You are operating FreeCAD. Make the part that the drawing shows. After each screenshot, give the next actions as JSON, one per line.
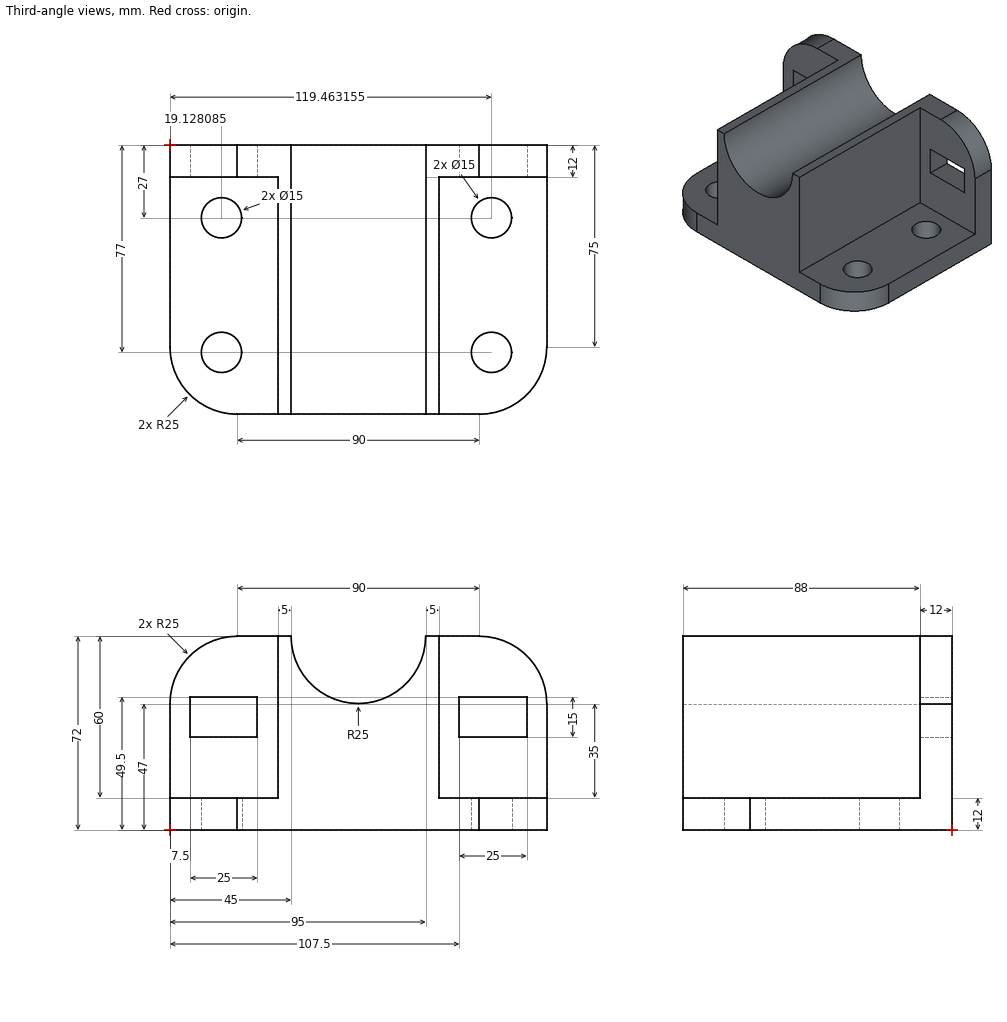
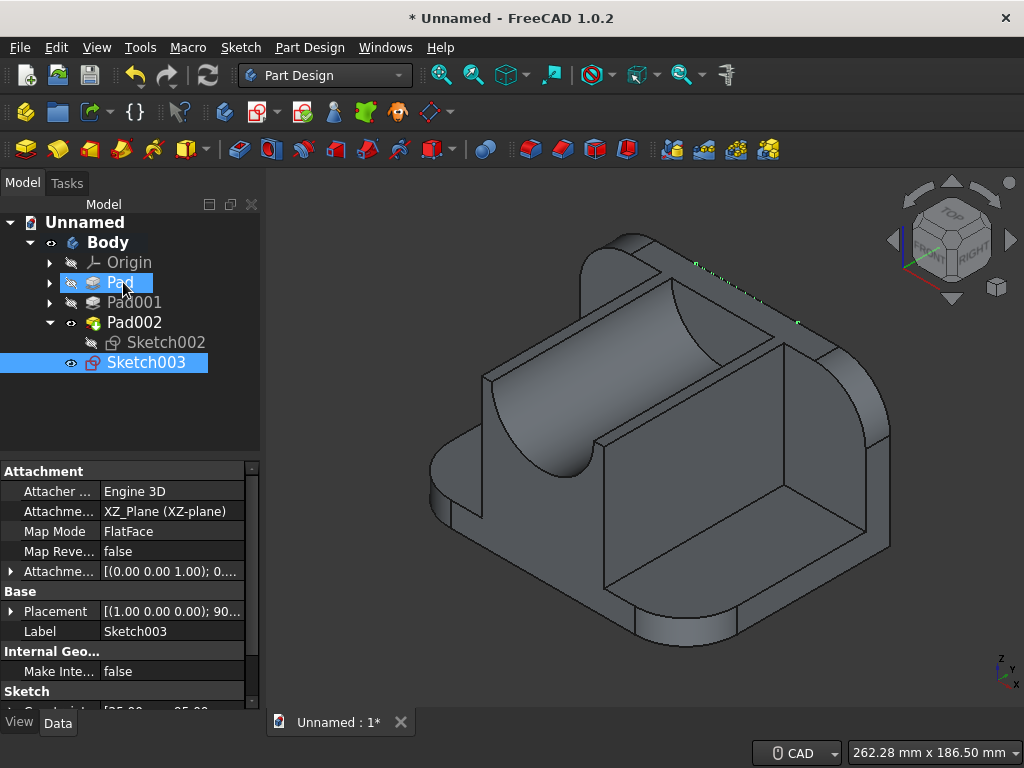
{"action": "left_click", "coordinate": [240, 150]}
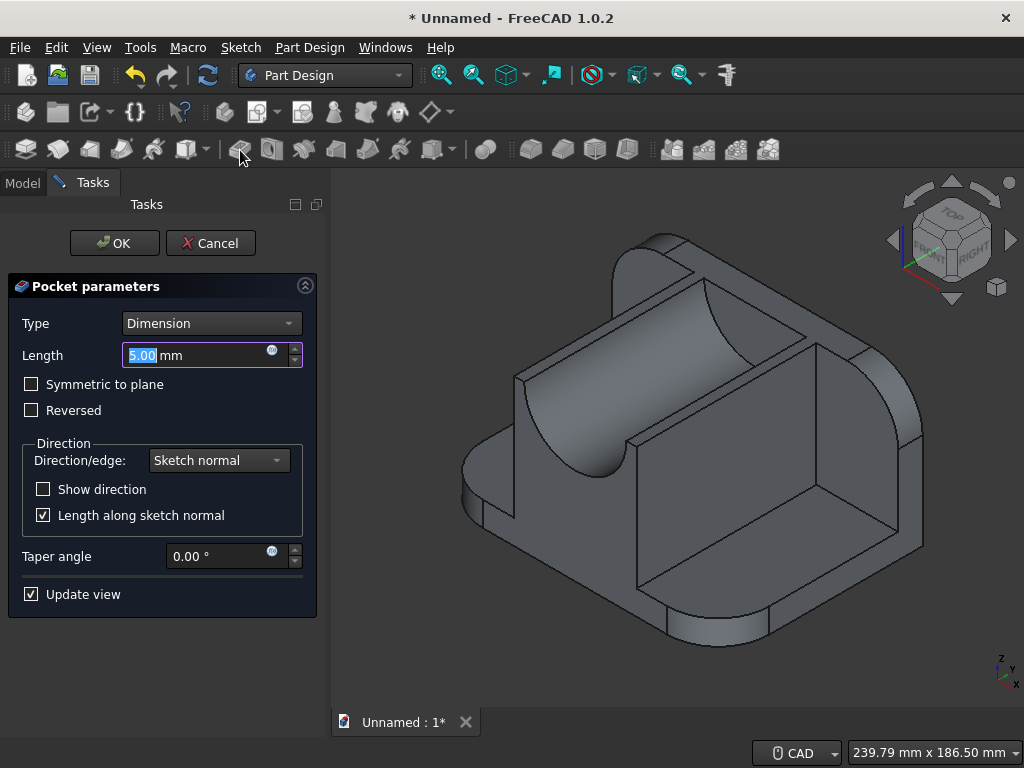
{"action": "type", "text": "12"}
{"action": "key", "text": "Tab"}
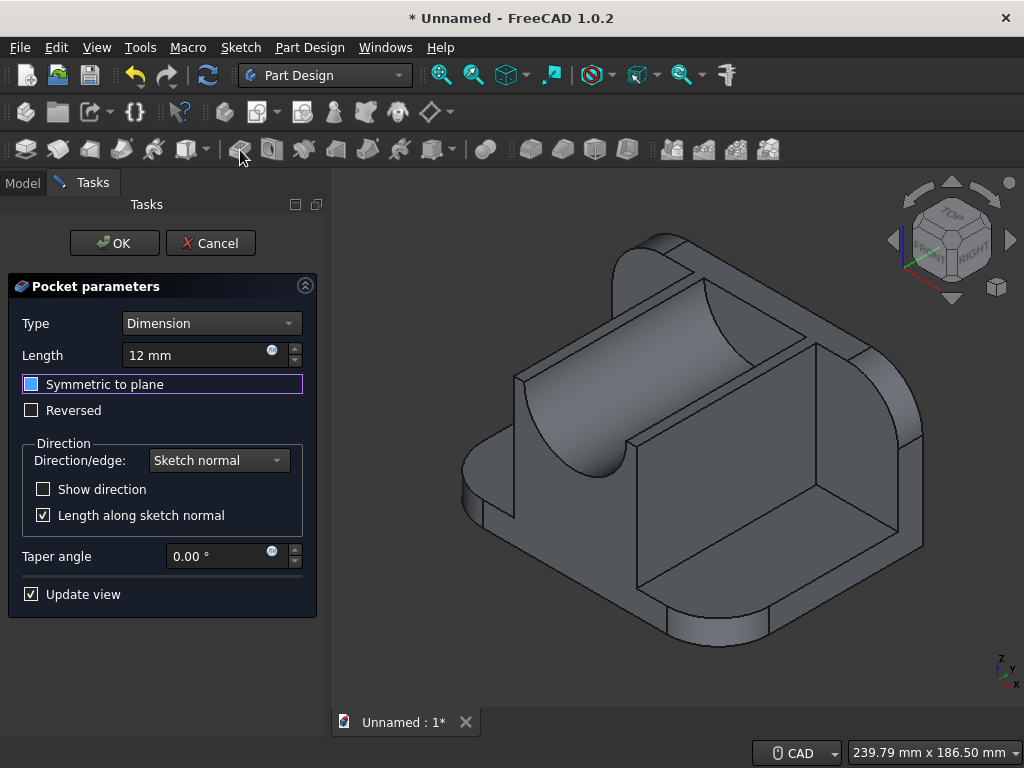
{"action": "left_click", "coordinate": [30, 410]}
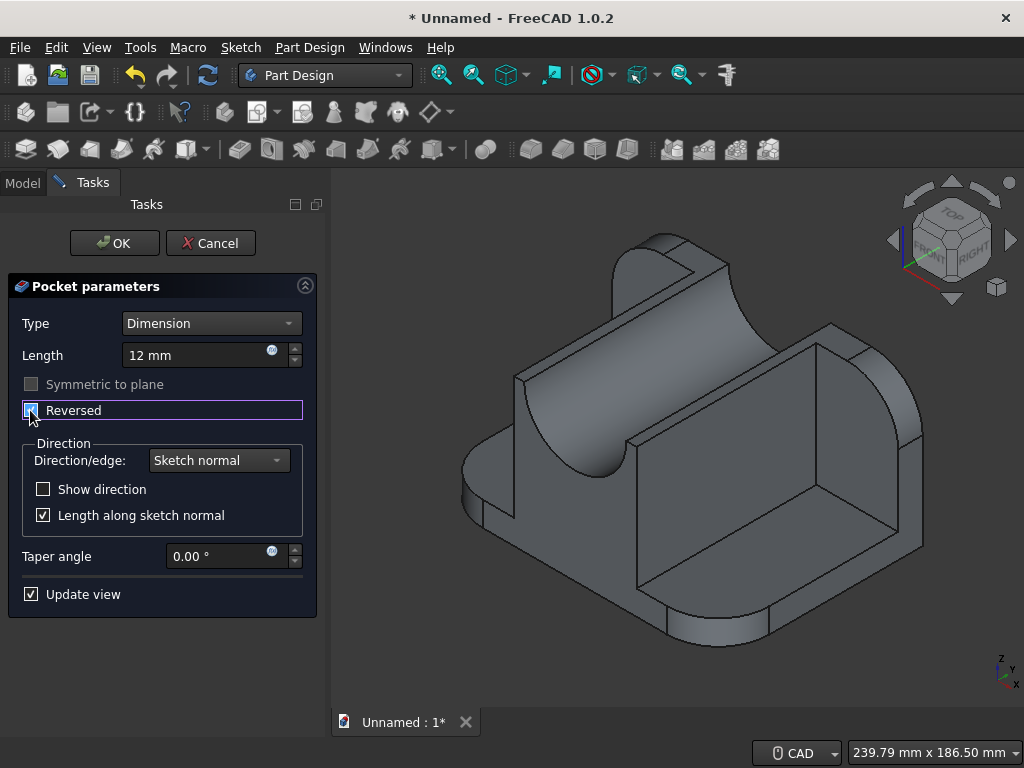
{"action": "left_click", "coordinate": [115, 243]}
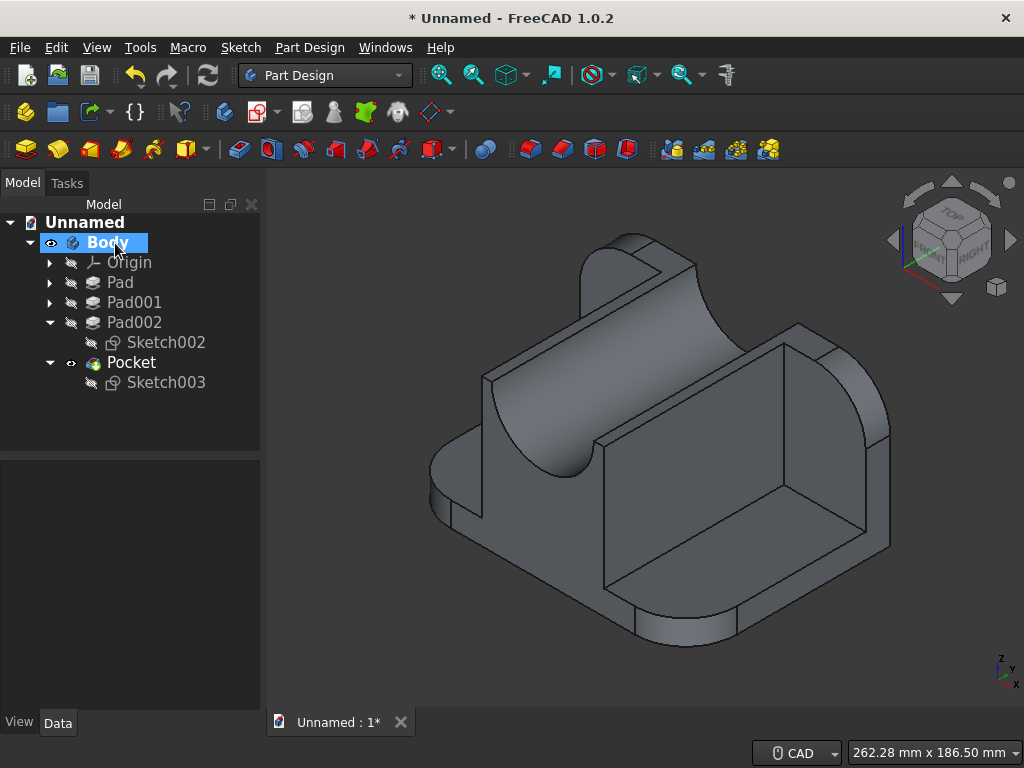
{"action": "key", "text": "1"}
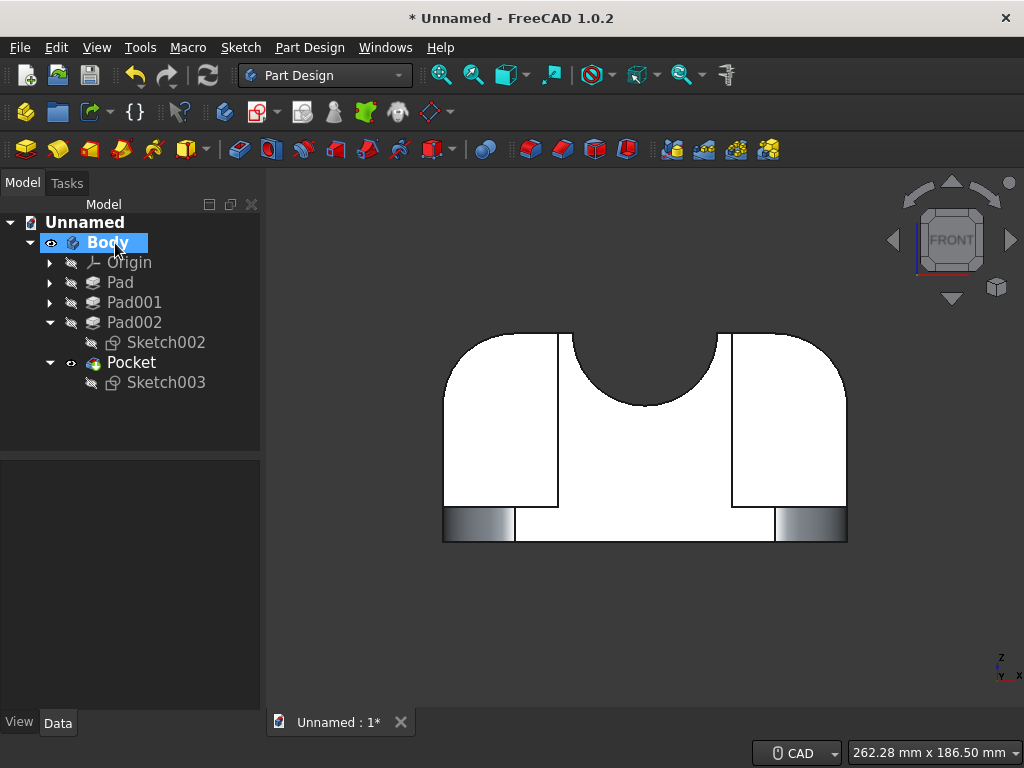
{"action": "left_click", "coordinate": [500, 419]}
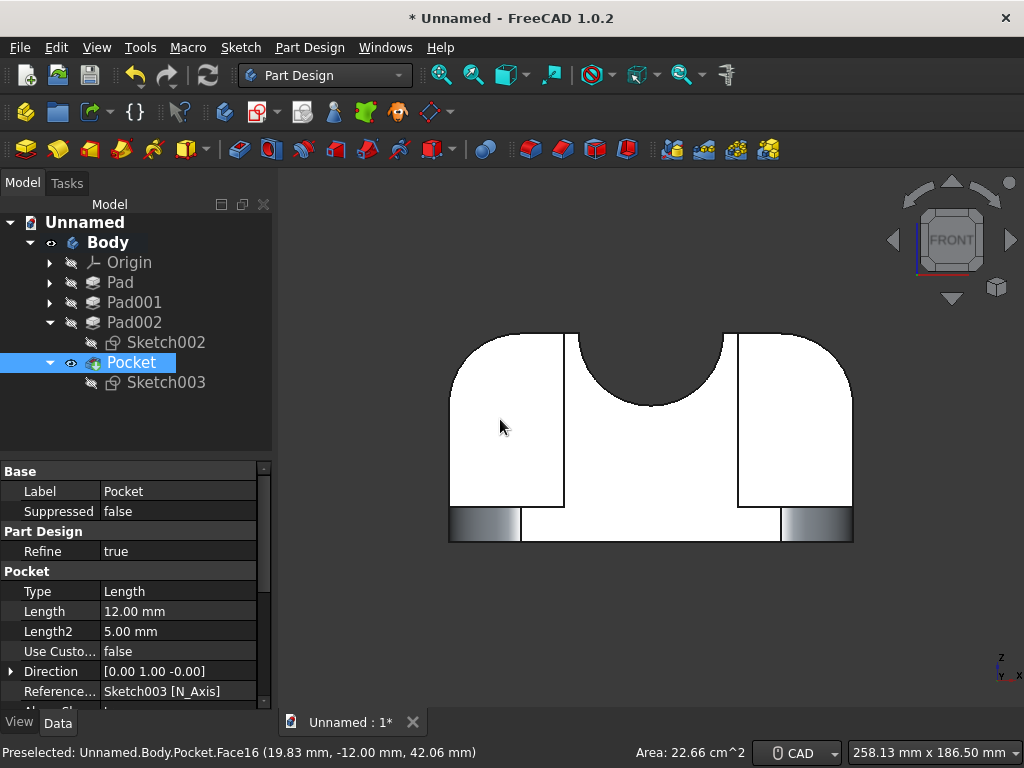
{"action": "left_click", "coordinate": [258, 112]}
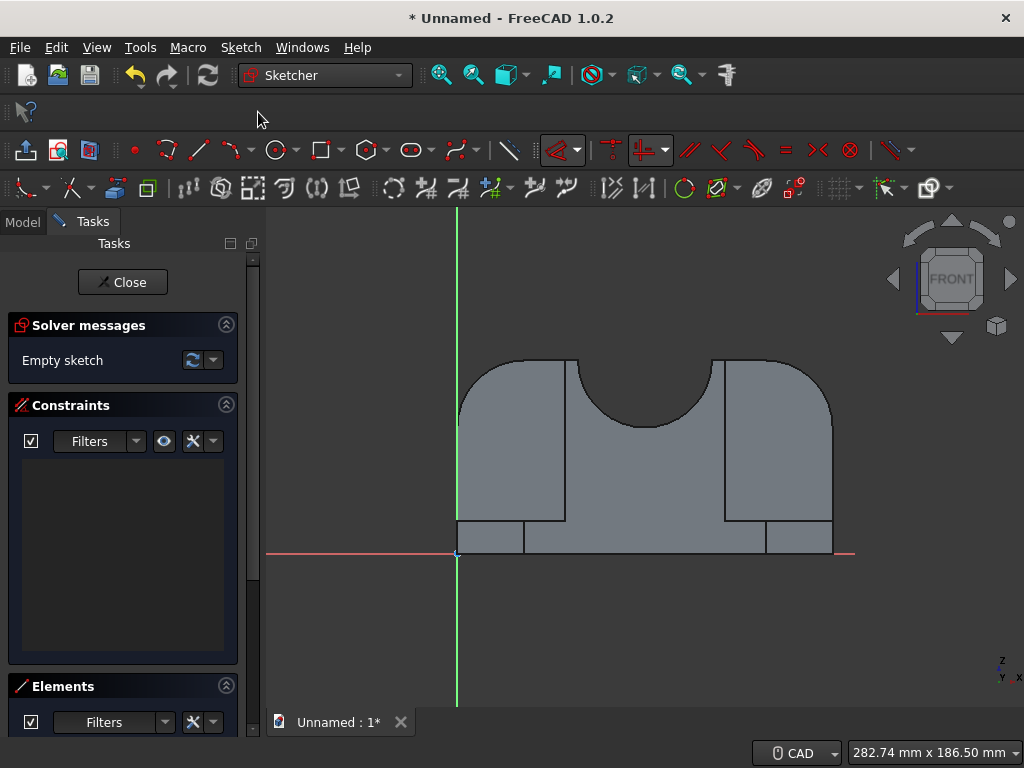
{"action": "scroll", "coordinate": [819, 438], "scroll_direction": "up", "scroll_amount": 9}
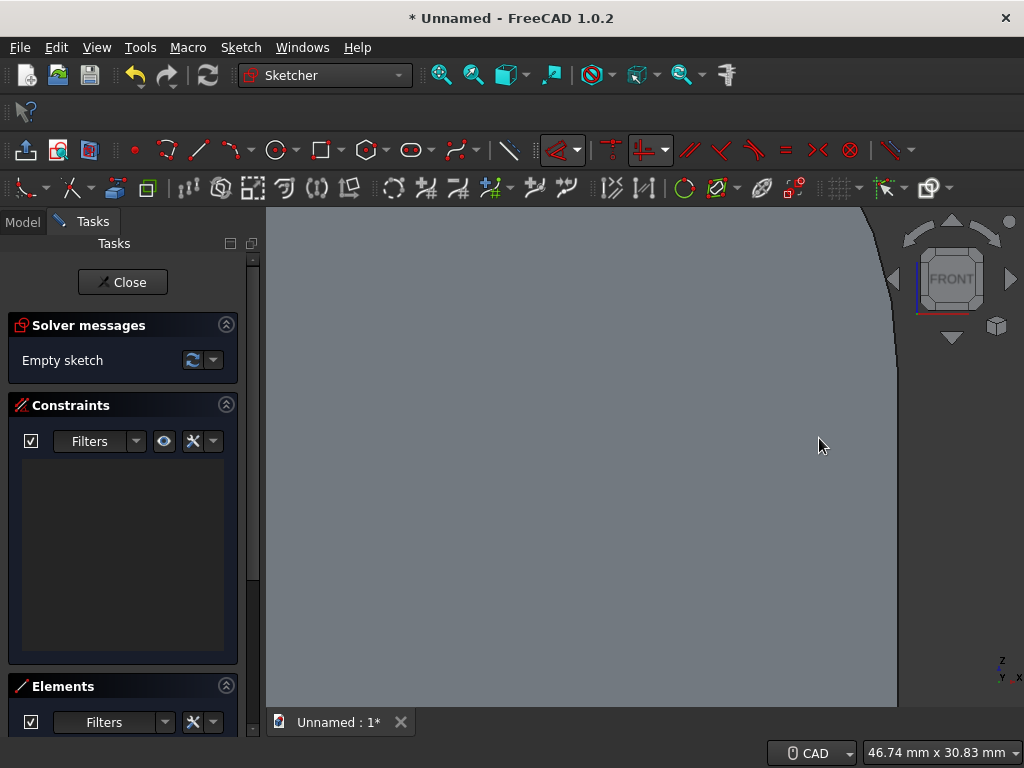
{"action": "key", "text": "g r"}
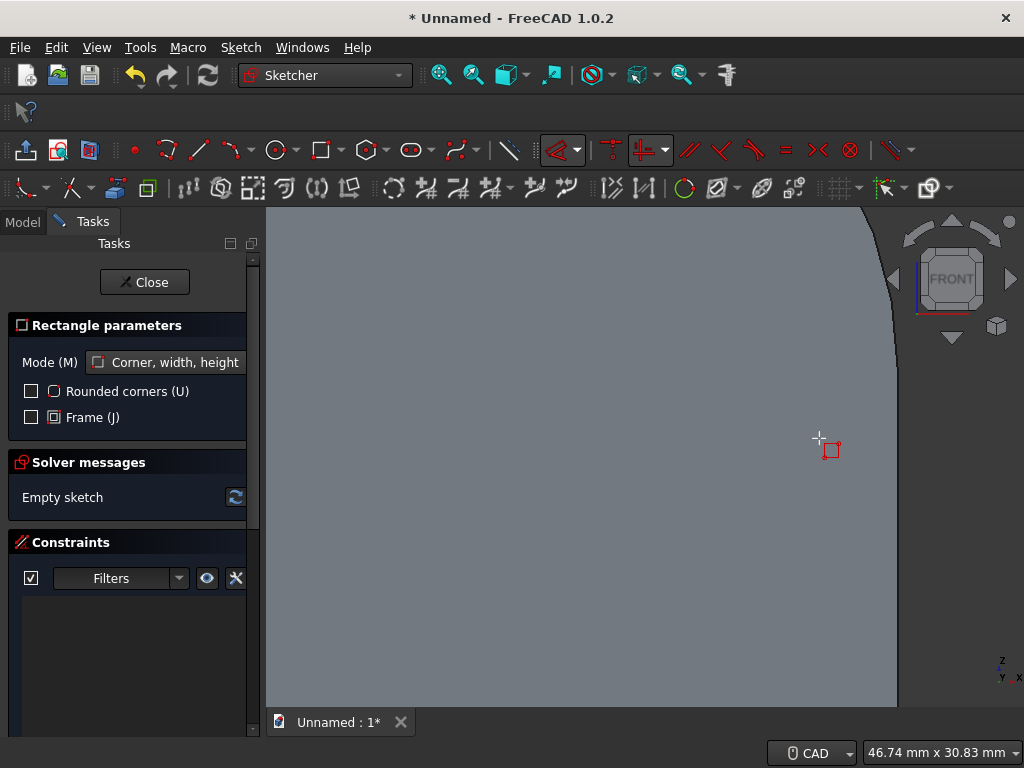
{"action": "left_click", "coordinate": [371, 332]}
{"action": "left_click", "coordinate": [776, 575]}
{"action": "key", "text": "Escape"}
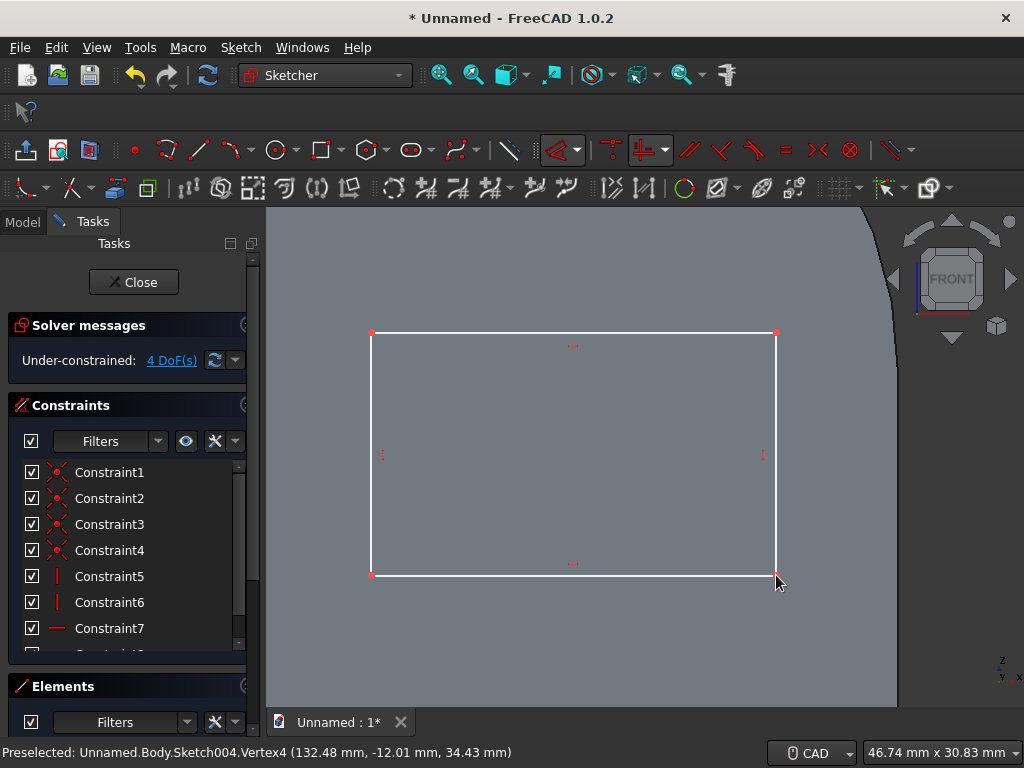
{"action": "left_click", "coordinate": [371, 406]}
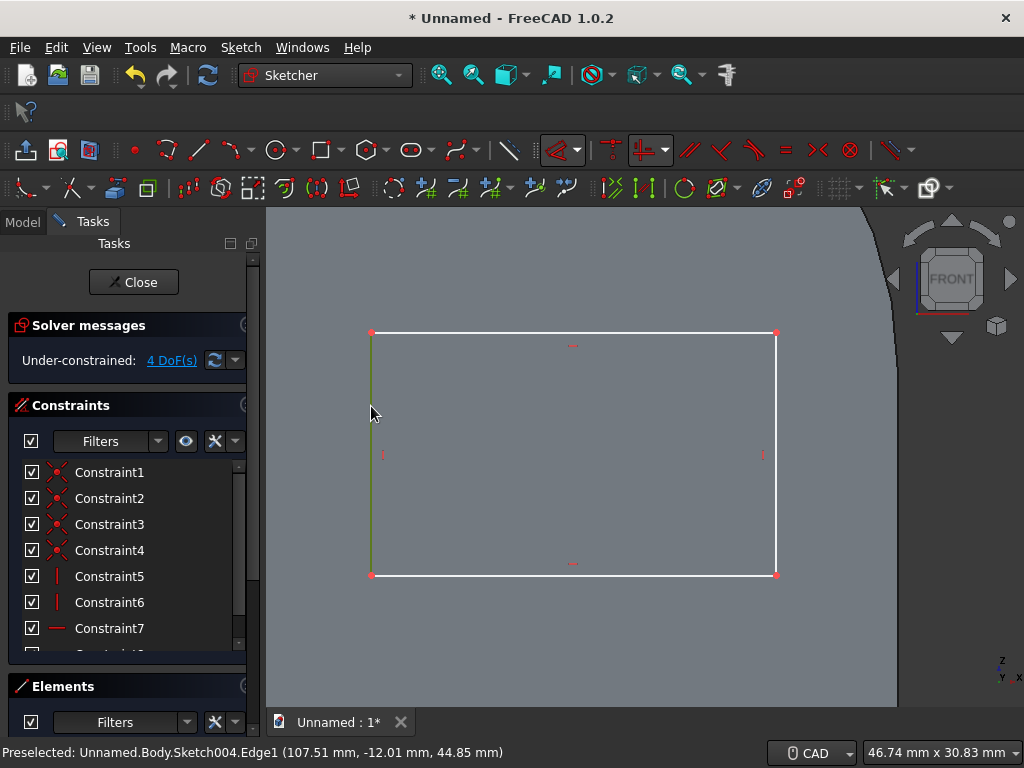
{"action": "key", "text": "i"}